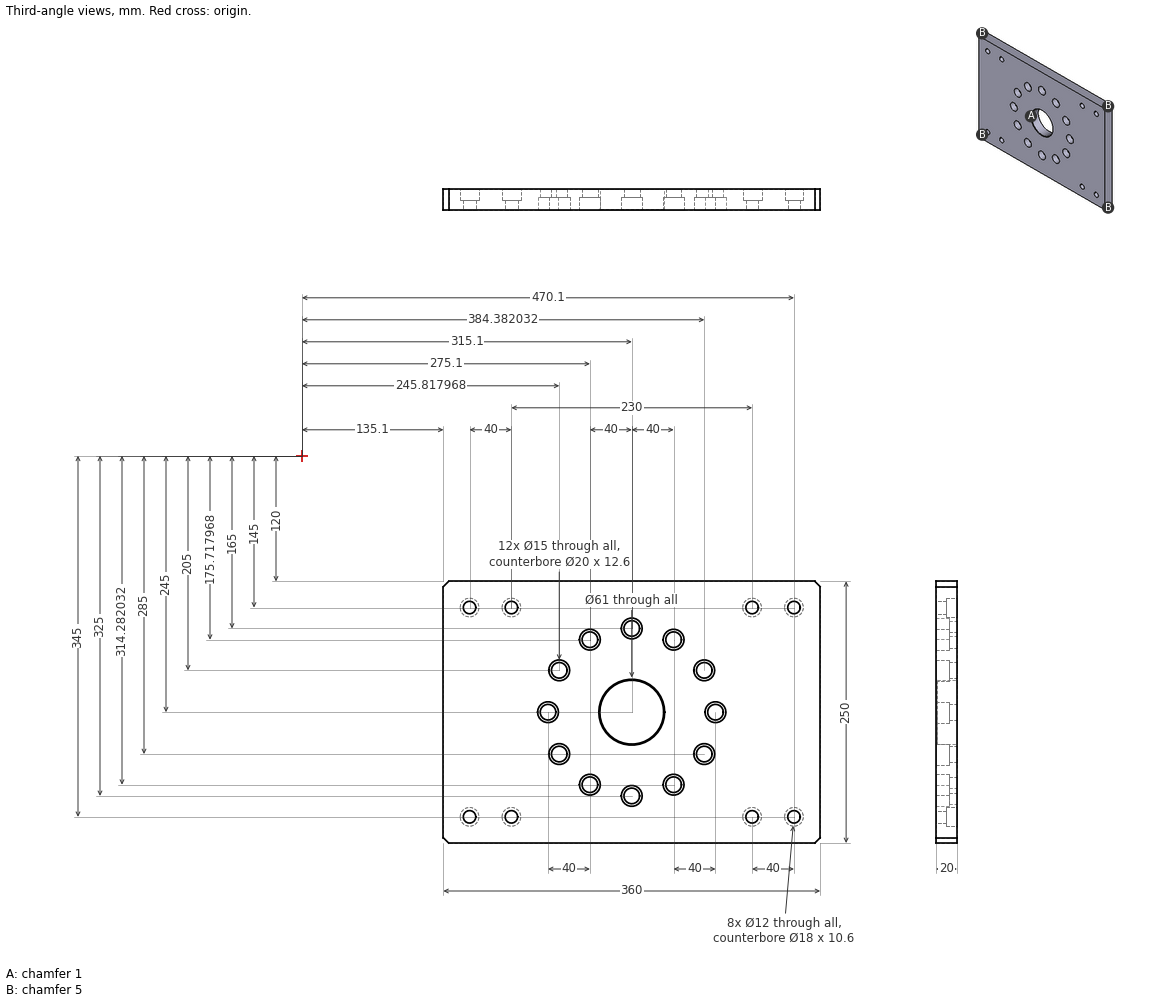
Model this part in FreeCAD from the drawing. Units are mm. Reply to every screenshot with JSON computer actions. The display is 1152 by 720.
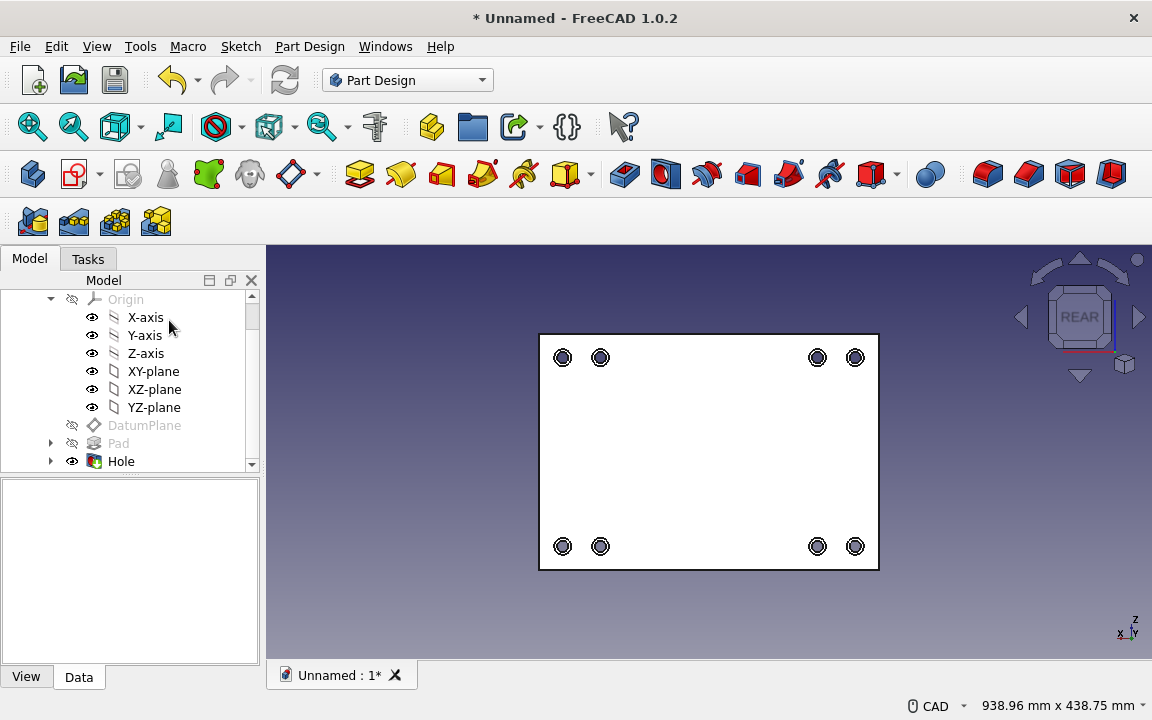
{"action": "key", "text": "0"}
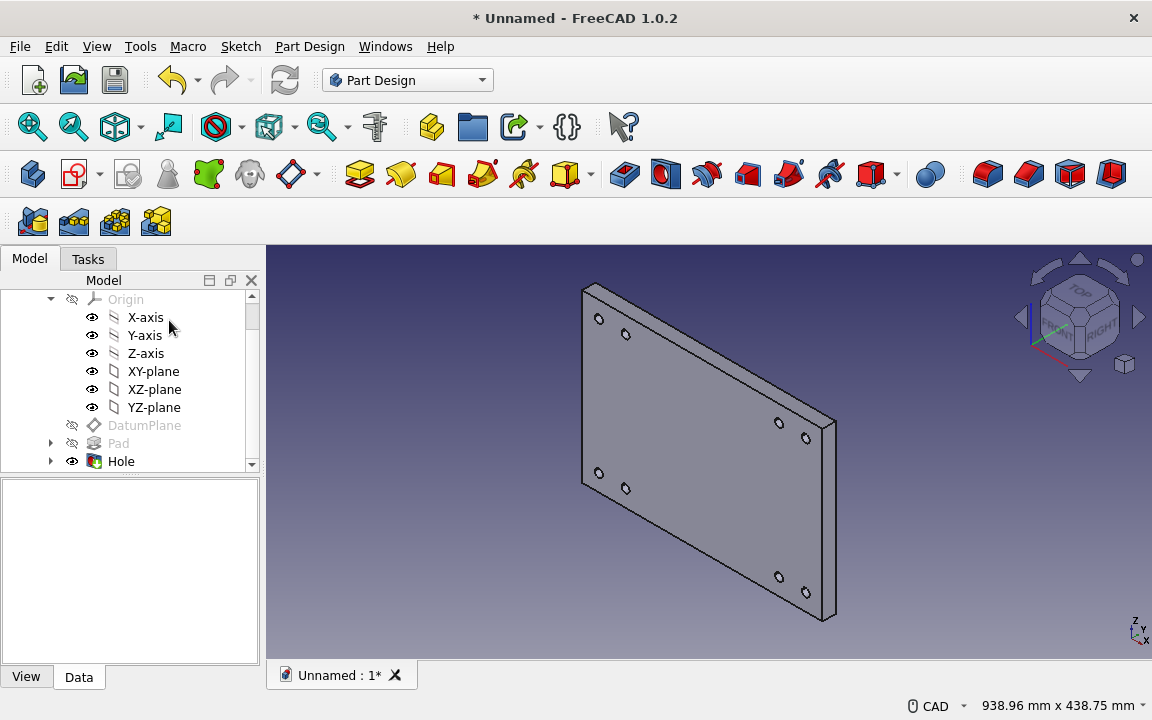
{"action": "left_click", "coordinate": [702, 455]}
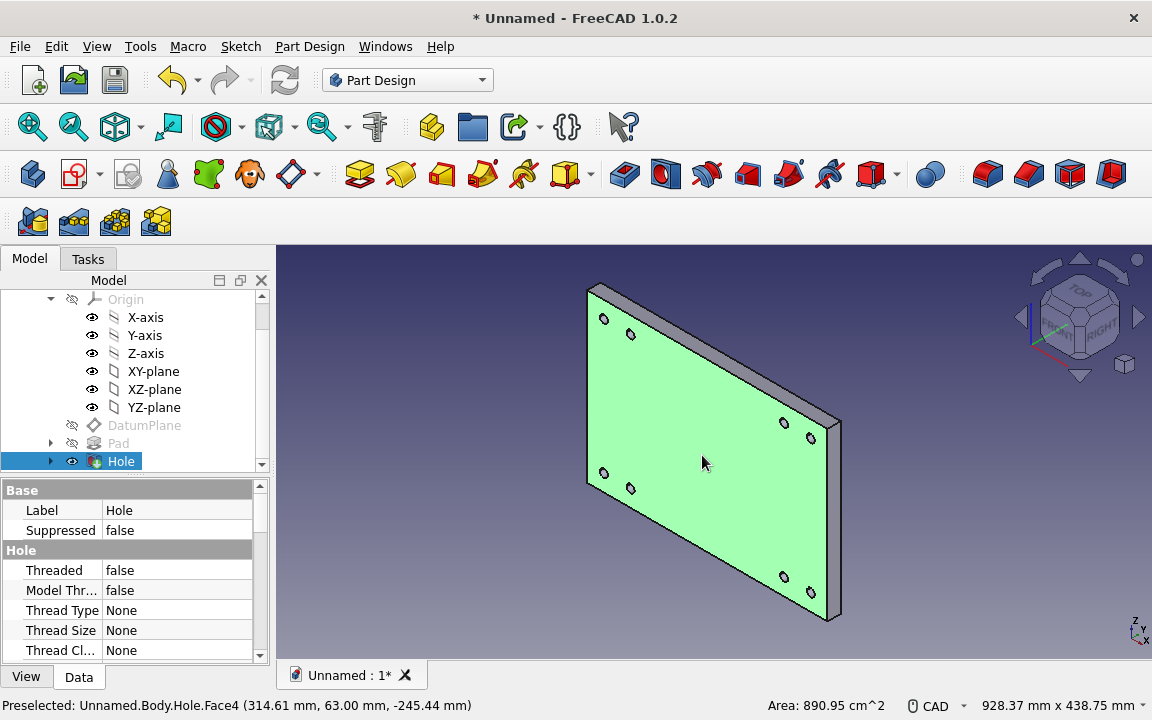
{"action": "left_click", "coordinate": [74, 174]}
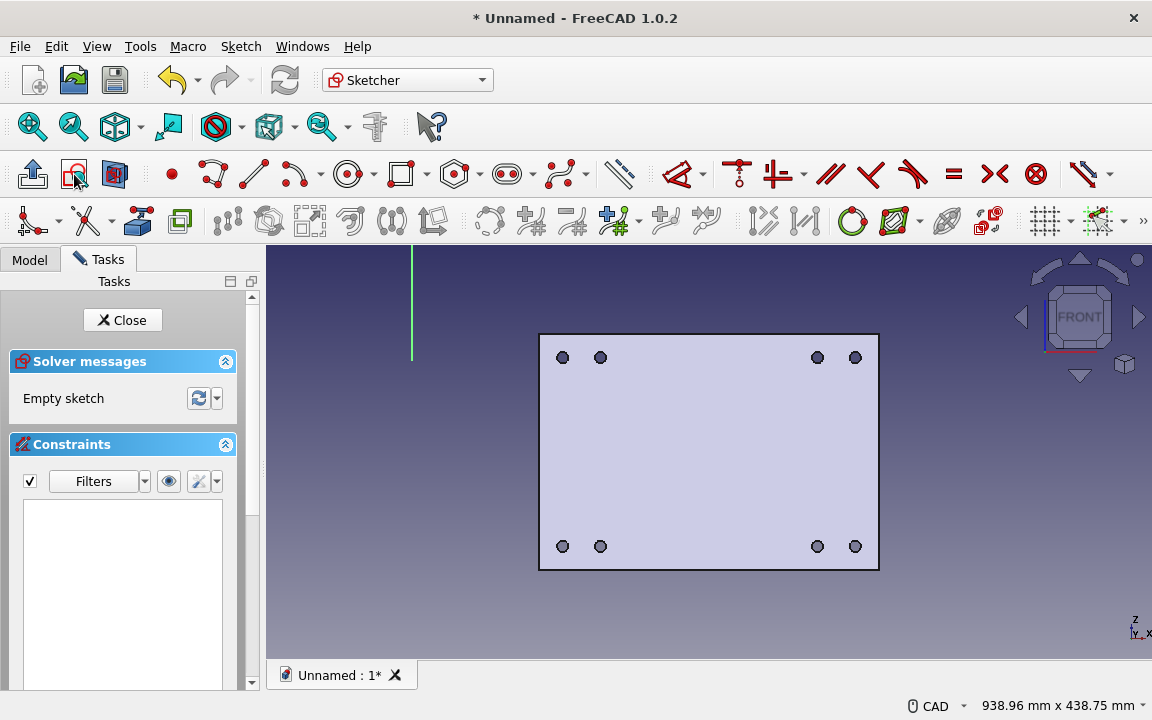
{"action": "scroll", "coordinate": [731, 452], "scroll_direction": "up", "scroll_amount": 7}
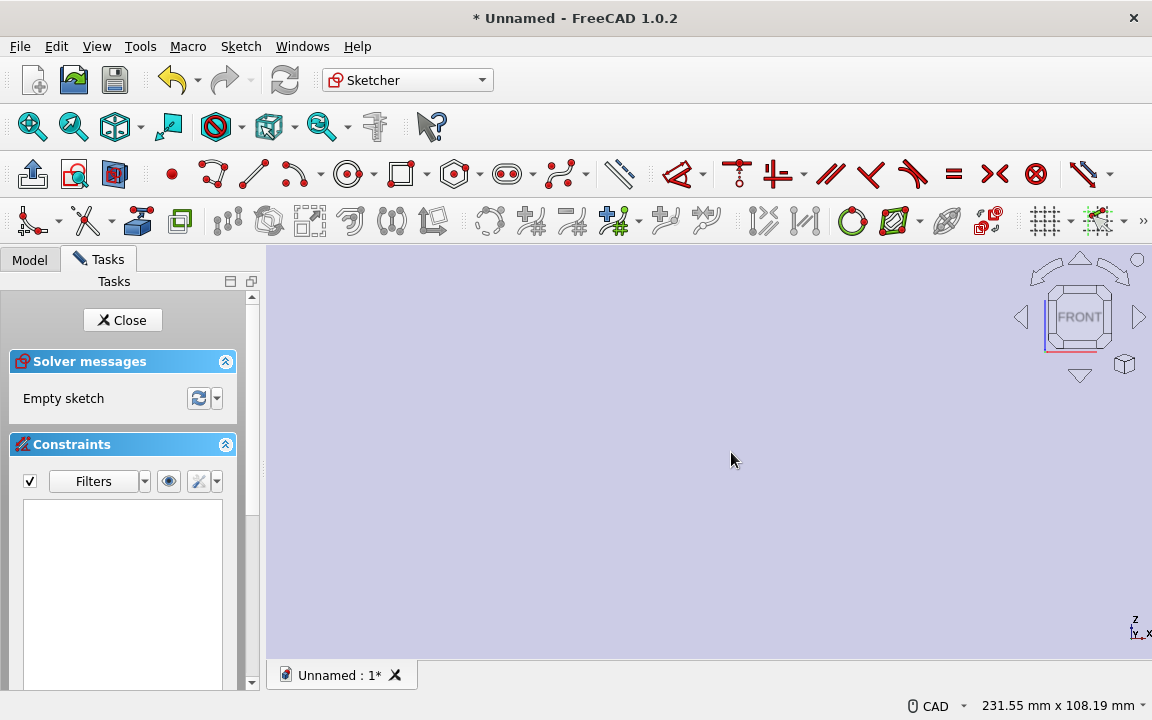
{"action": "left_click", "coordinate": [348, 174]}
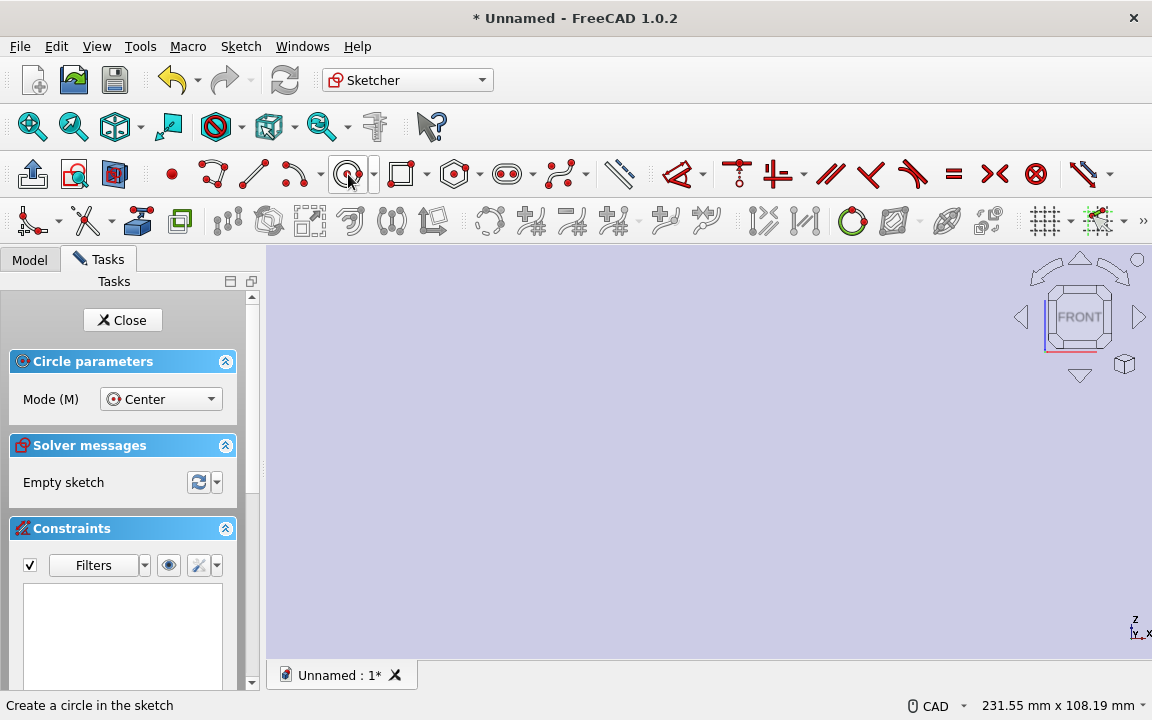
{"action": "left_click", "coordinate": [640, 450]}
{"action": "mouse_move", "coordinate": [723, 368]}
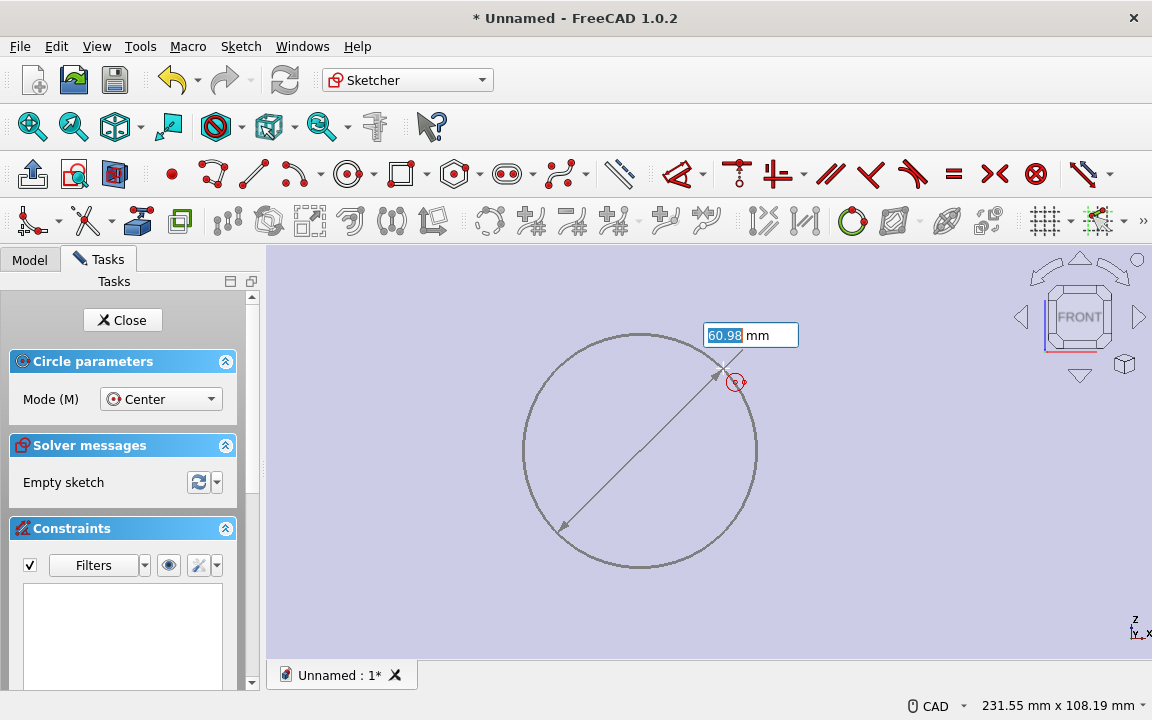
{"action": "type", "text": "61"}
{"action": "key", "text": "Return"}
{"action": "key", "text": "Escape"}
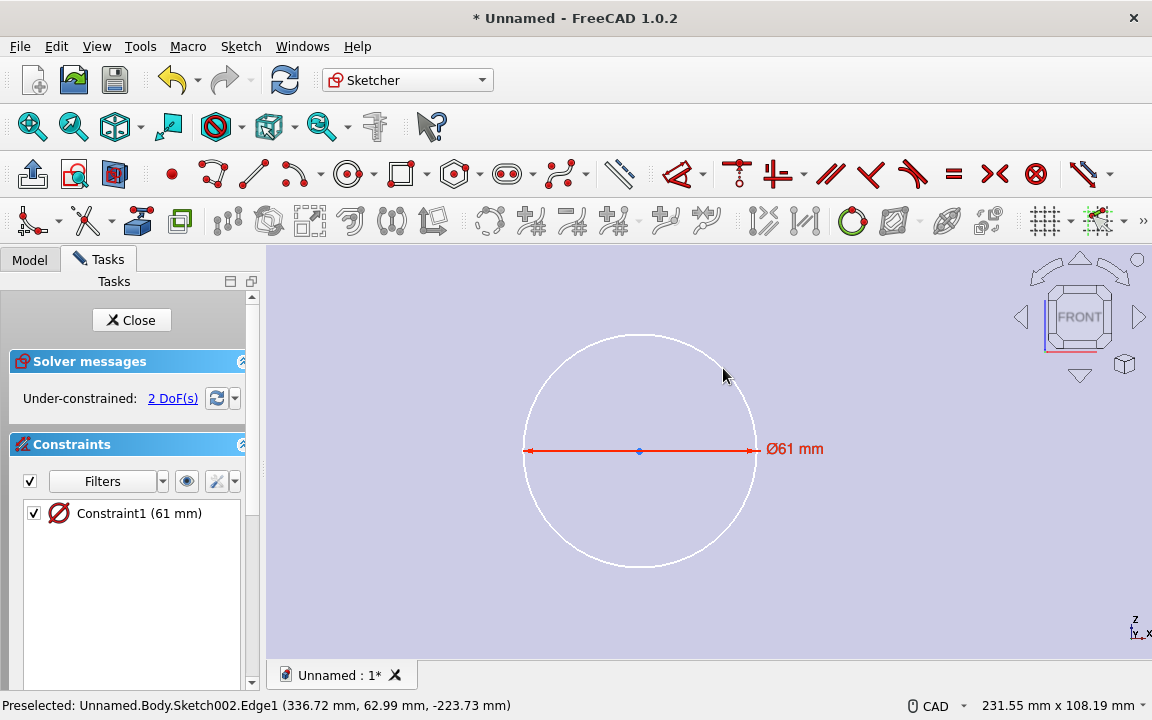
{"action": "left_click", "coordinate": [676, 174]}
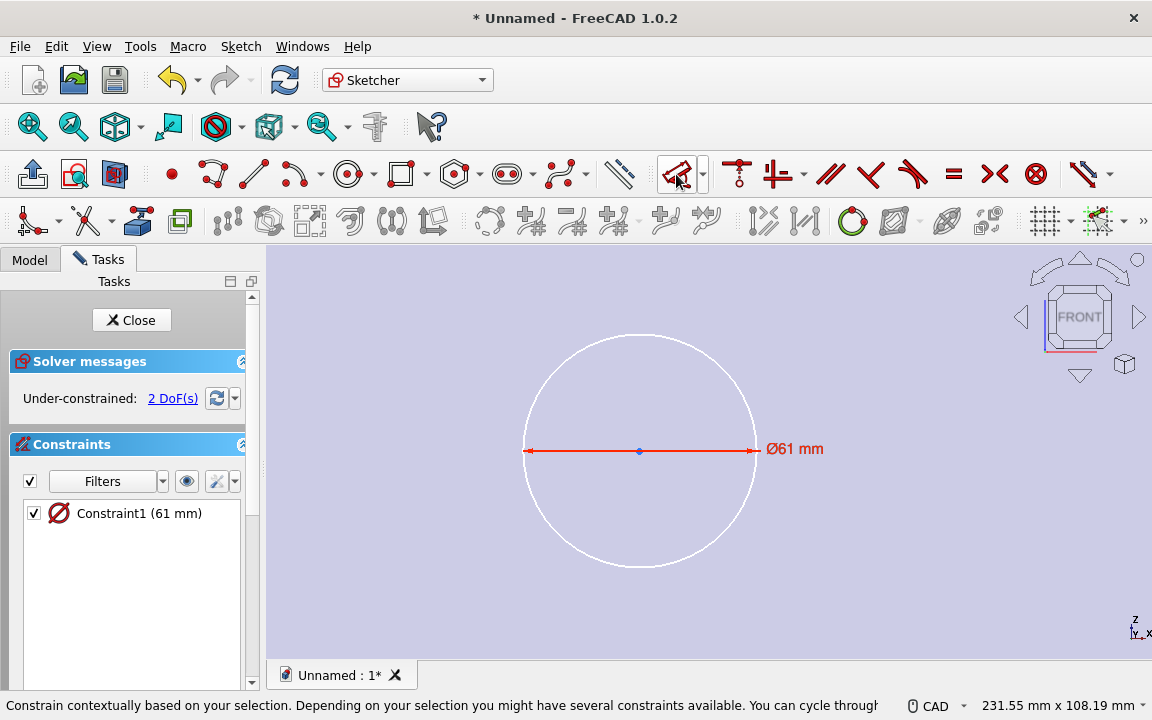
{"action": "left_click", "coordinate": [640, 451]}
{"action": "left_click", "coordinate": [674, 362]}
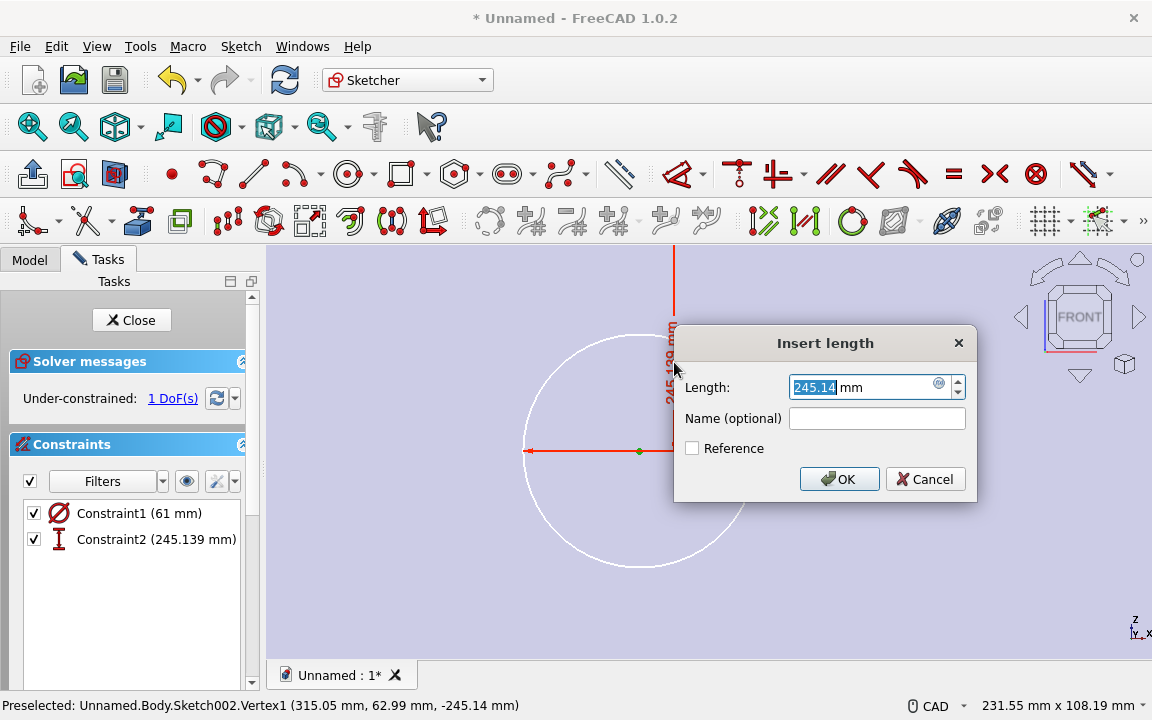
{"action": "type", "text": "245"}
{"action": "key", "text": "Return"}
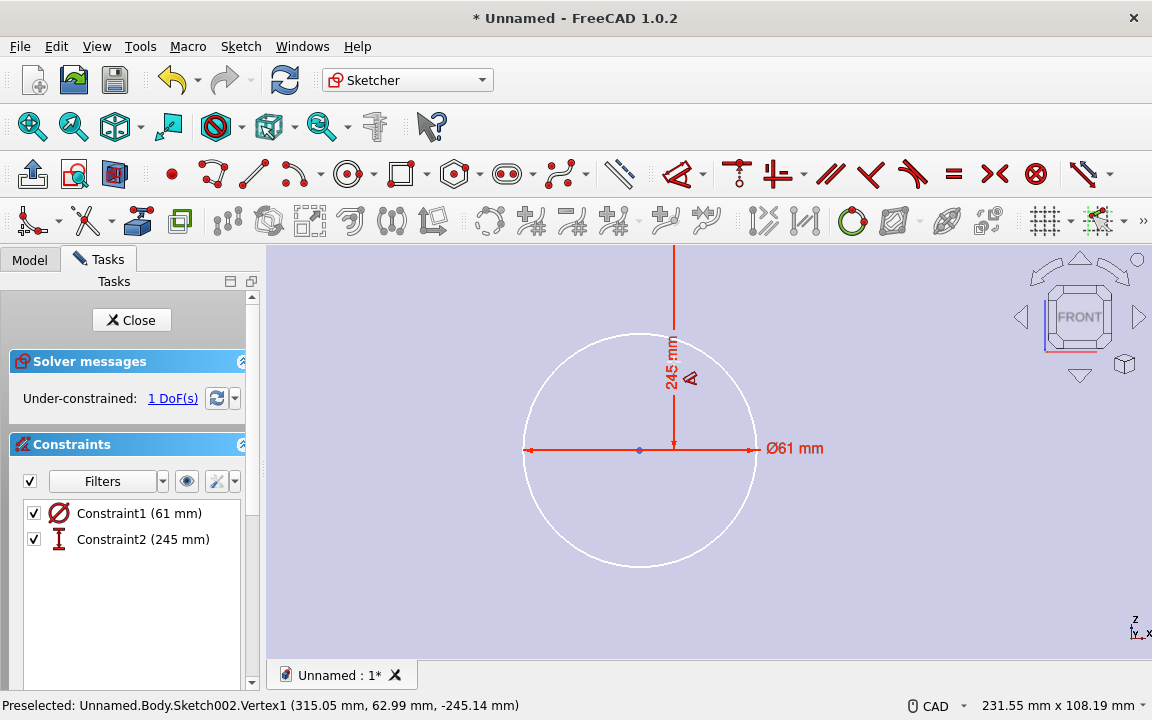
{"action": "left_click", "coordinate": [640, 450]}
{"action": "left_click", "coordinate": [467, 484]}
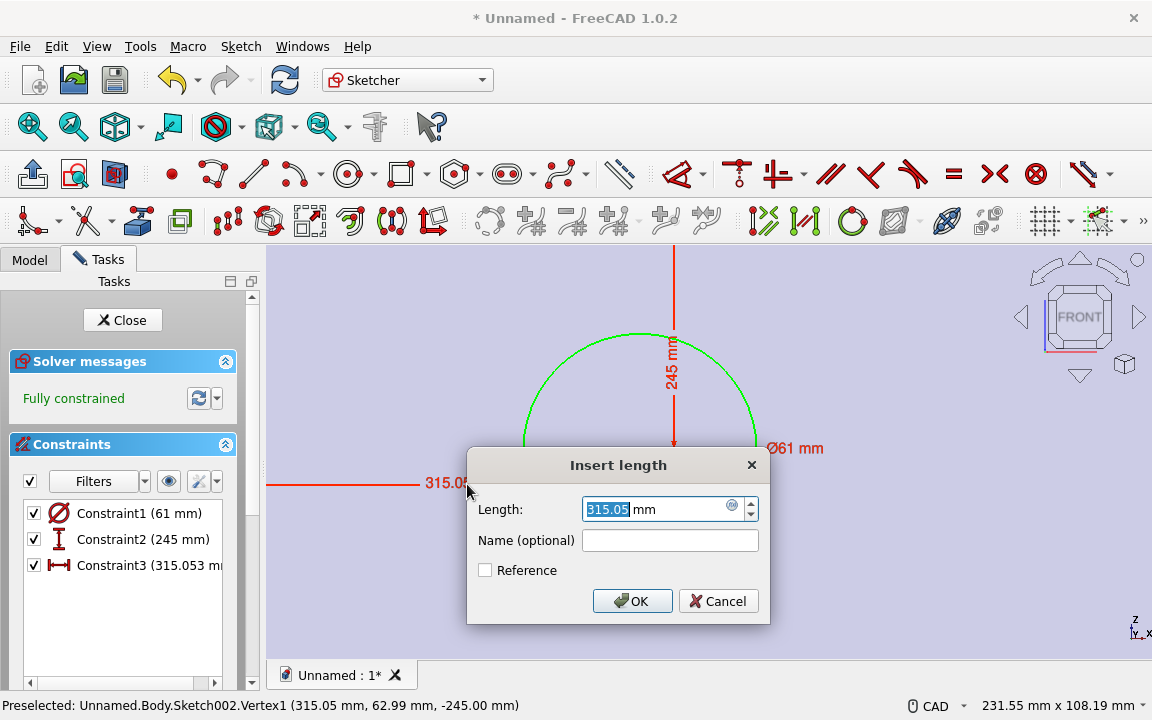
{"action": "type", "text": "315.1"}
{"action": "key", "text": "Return"}
{"action": "key", "text": "Escape"}